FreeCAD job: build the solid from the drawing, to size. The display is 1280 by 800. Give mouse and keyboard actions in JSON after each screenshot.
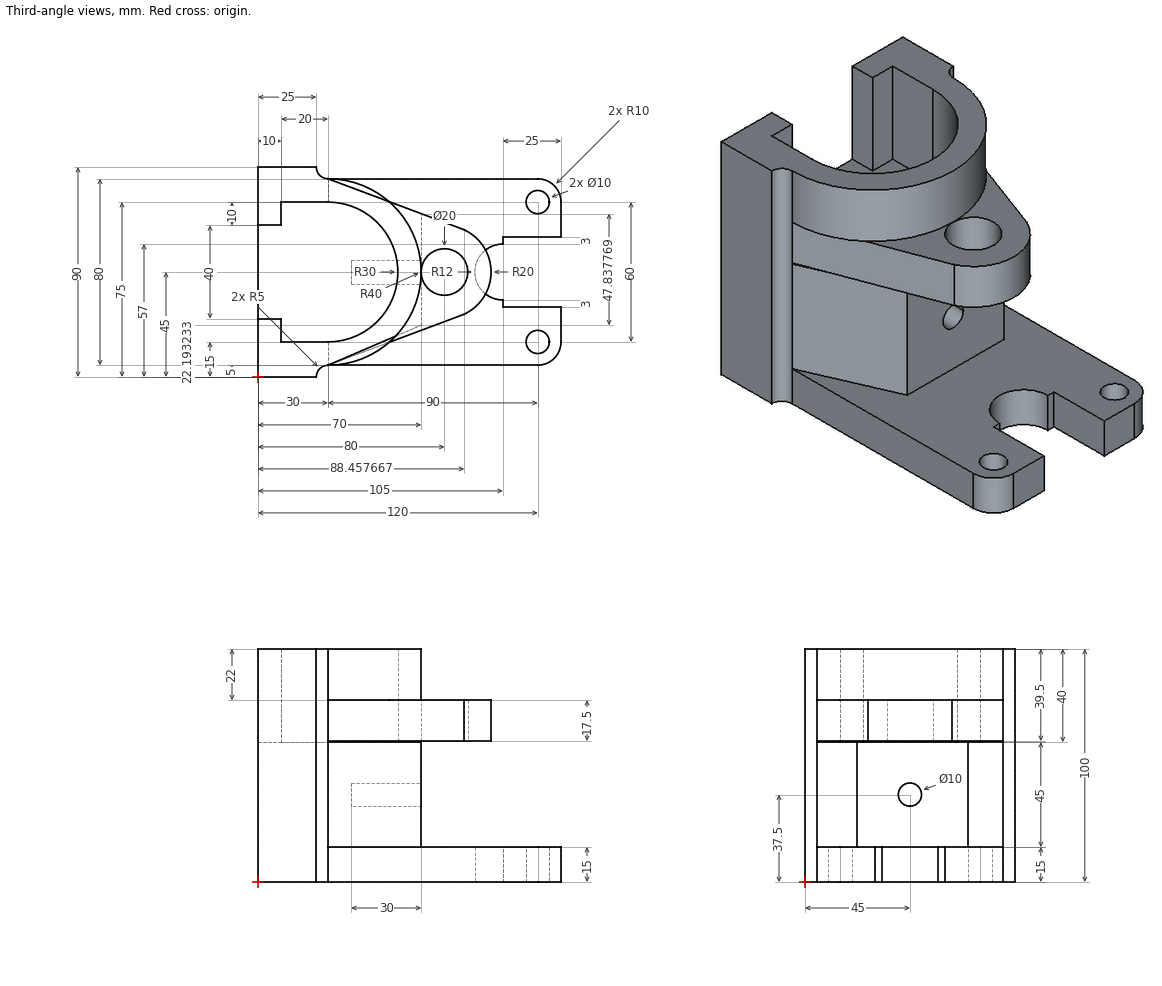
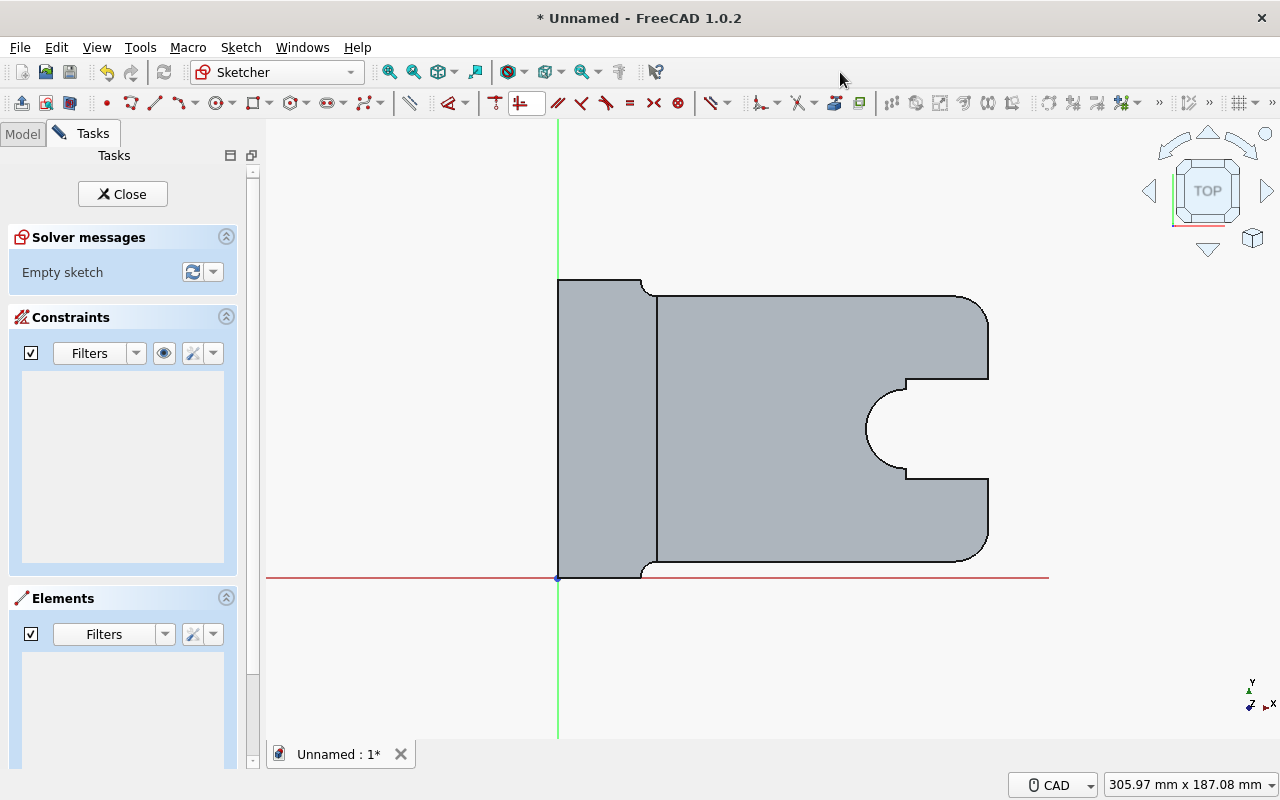
{"action": "scroll", "coordinate": [887, 479], "scroll_direction": "up", "scroll_amount": 2}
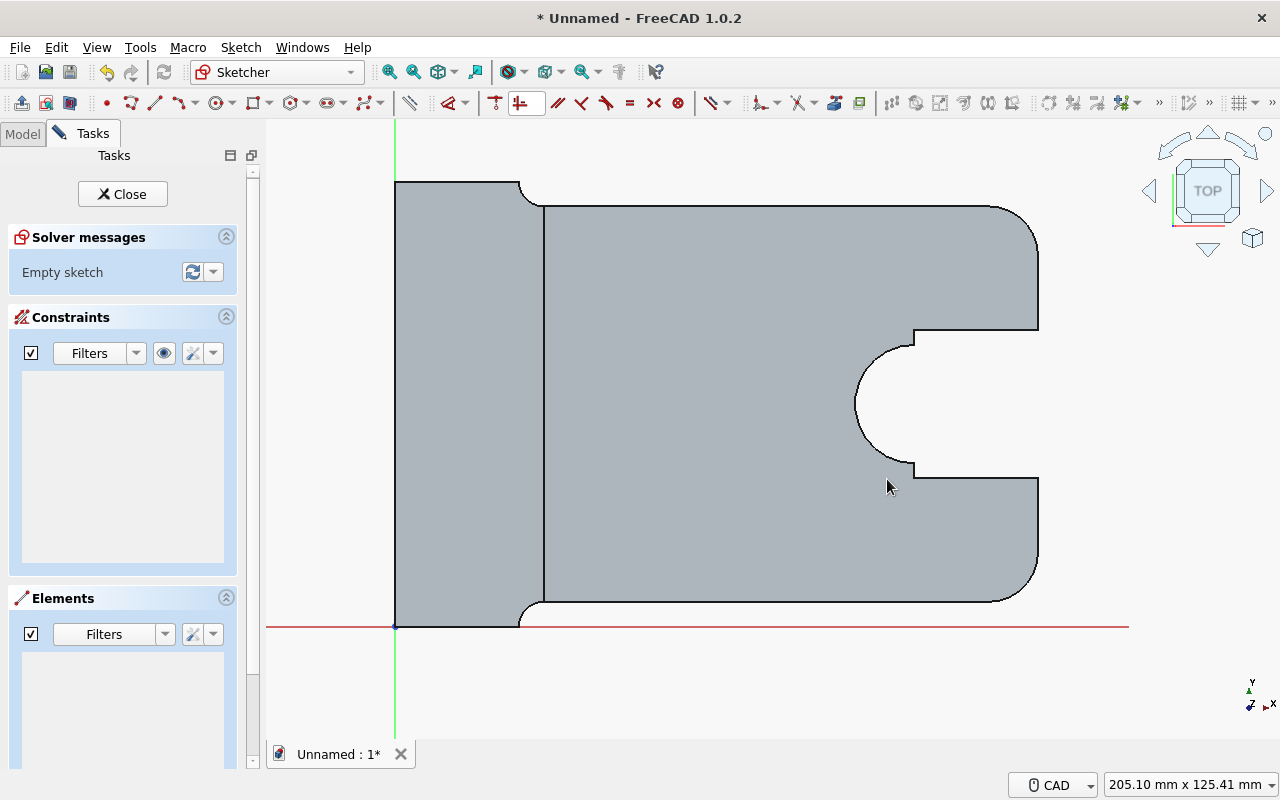
{"action": "left_click", "coordinate": [216, 104]}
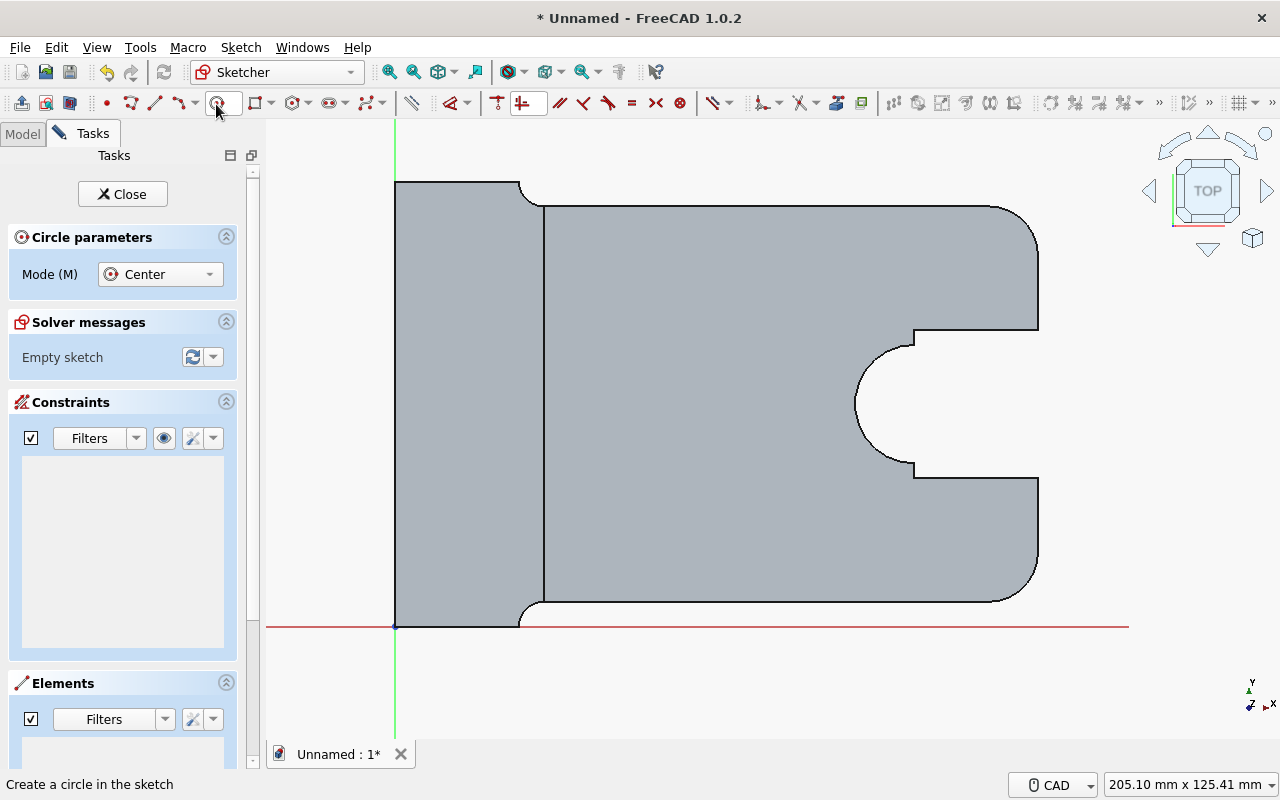
{"action": "left_click", "coordinate": [989, 256]}
{"action": "left_click", "coordinate": [1006, 238]}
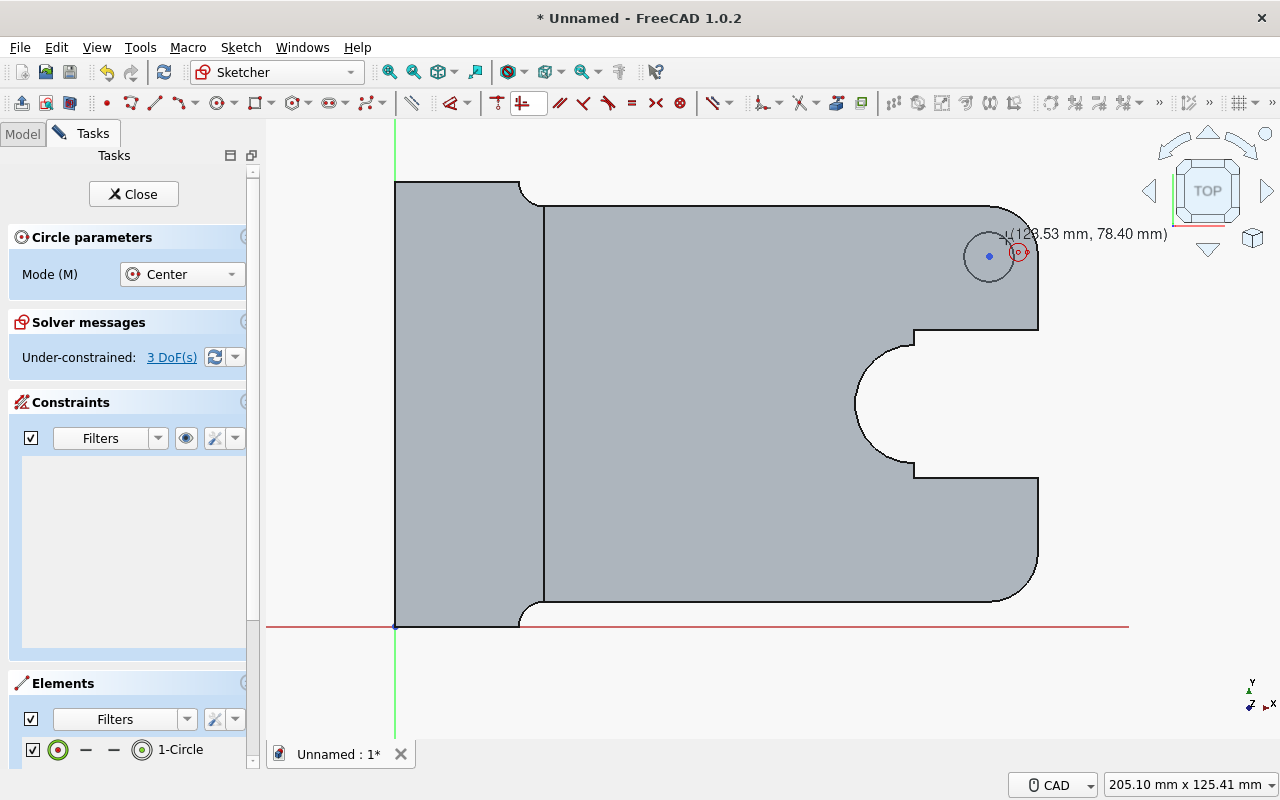
{"action": "left_click", "coordinate": [989, 552]}
{"action": "left_click", "coordinate": [1006, 535]}
{"action": "key", "text": "Escape"}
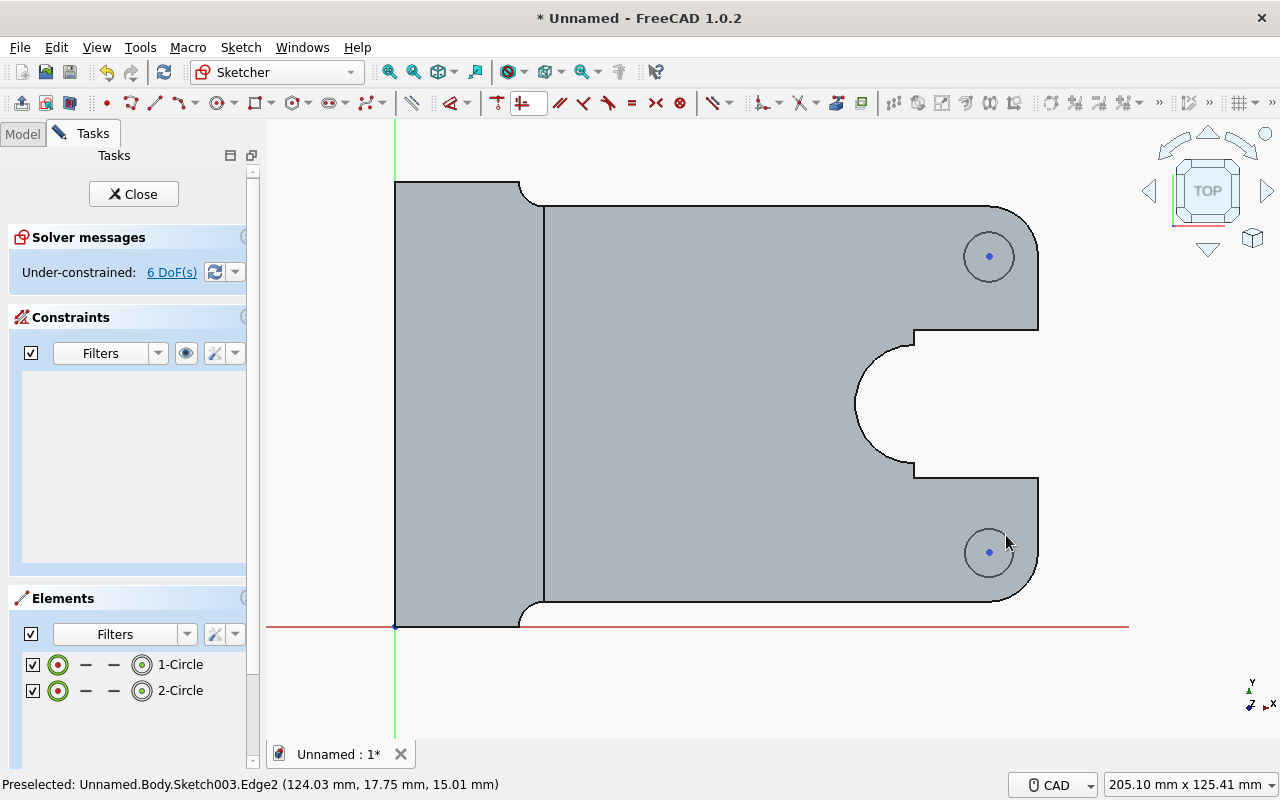
{"action": "left_click", "coordinate": [1006, 239]}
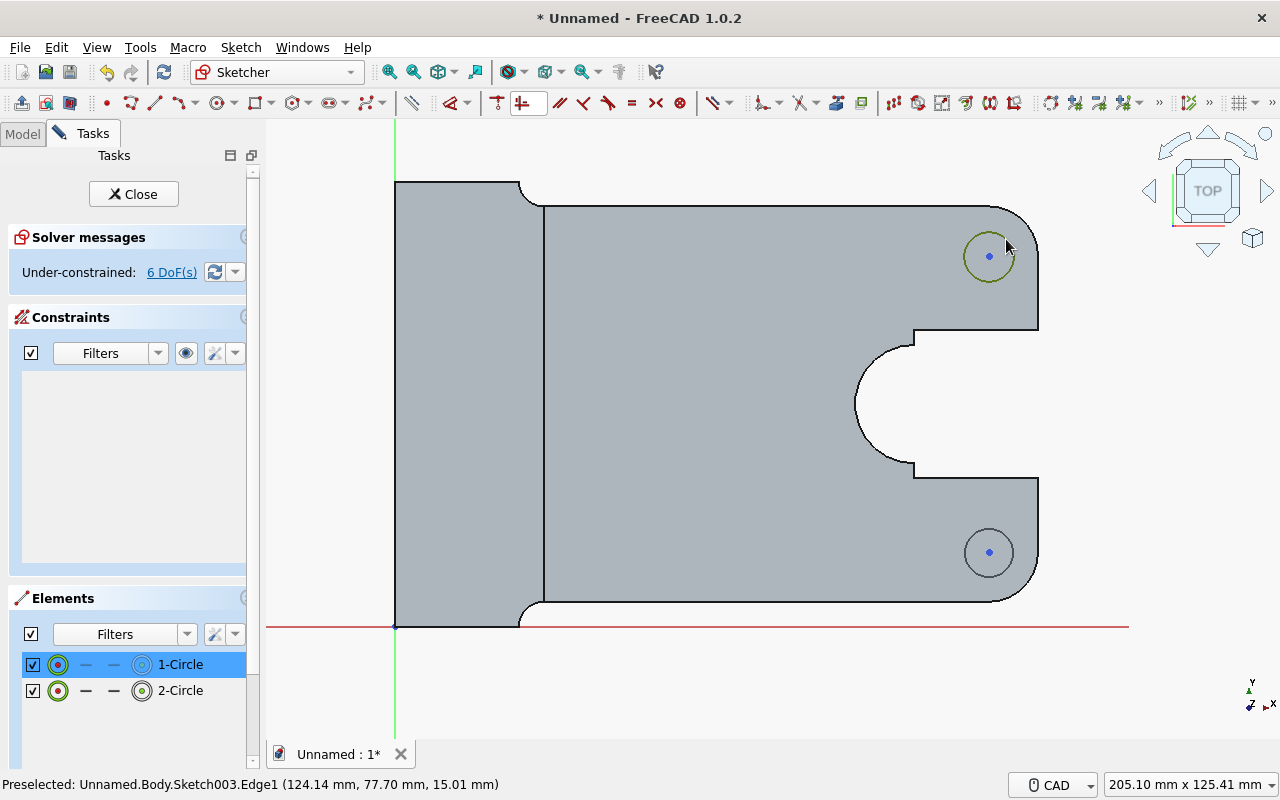
{"action": "left_click", "coordinate": [1006, 536]}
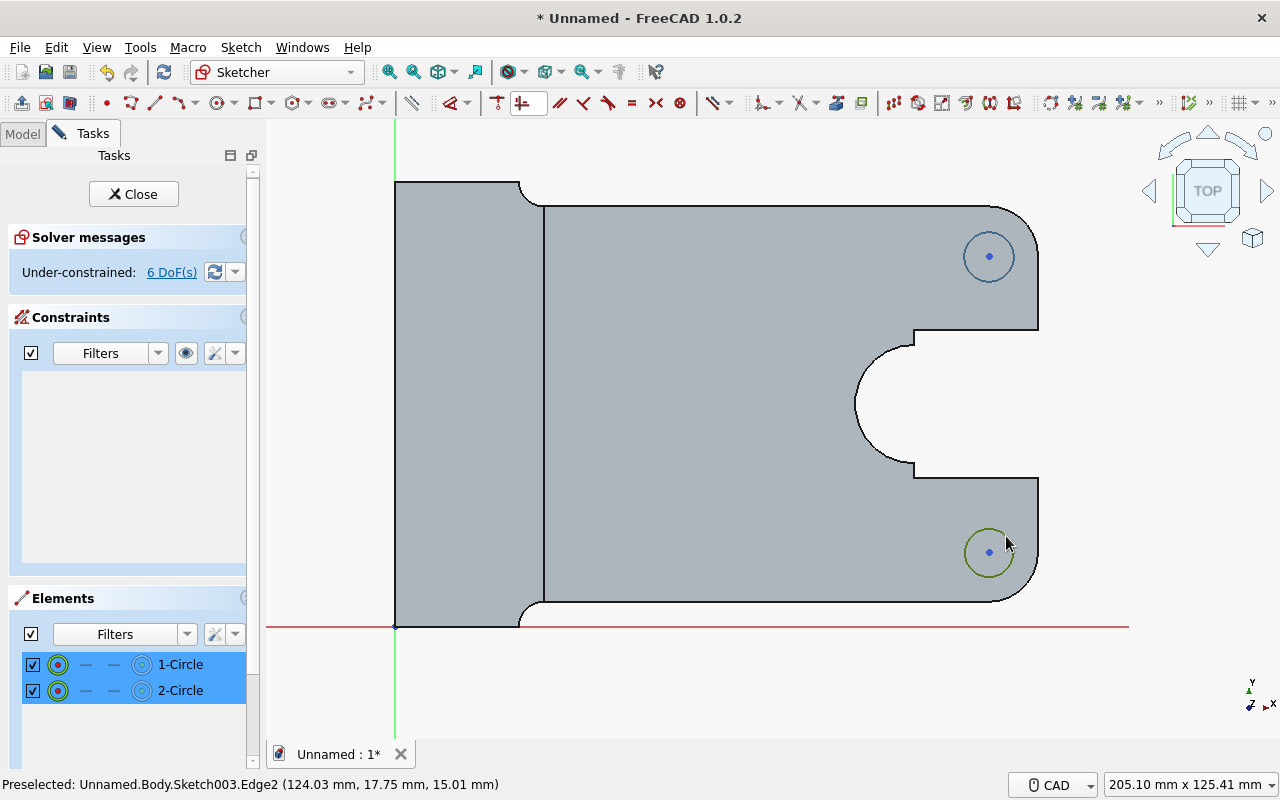
{"action": "left_click", "coordinate": [632, 104]}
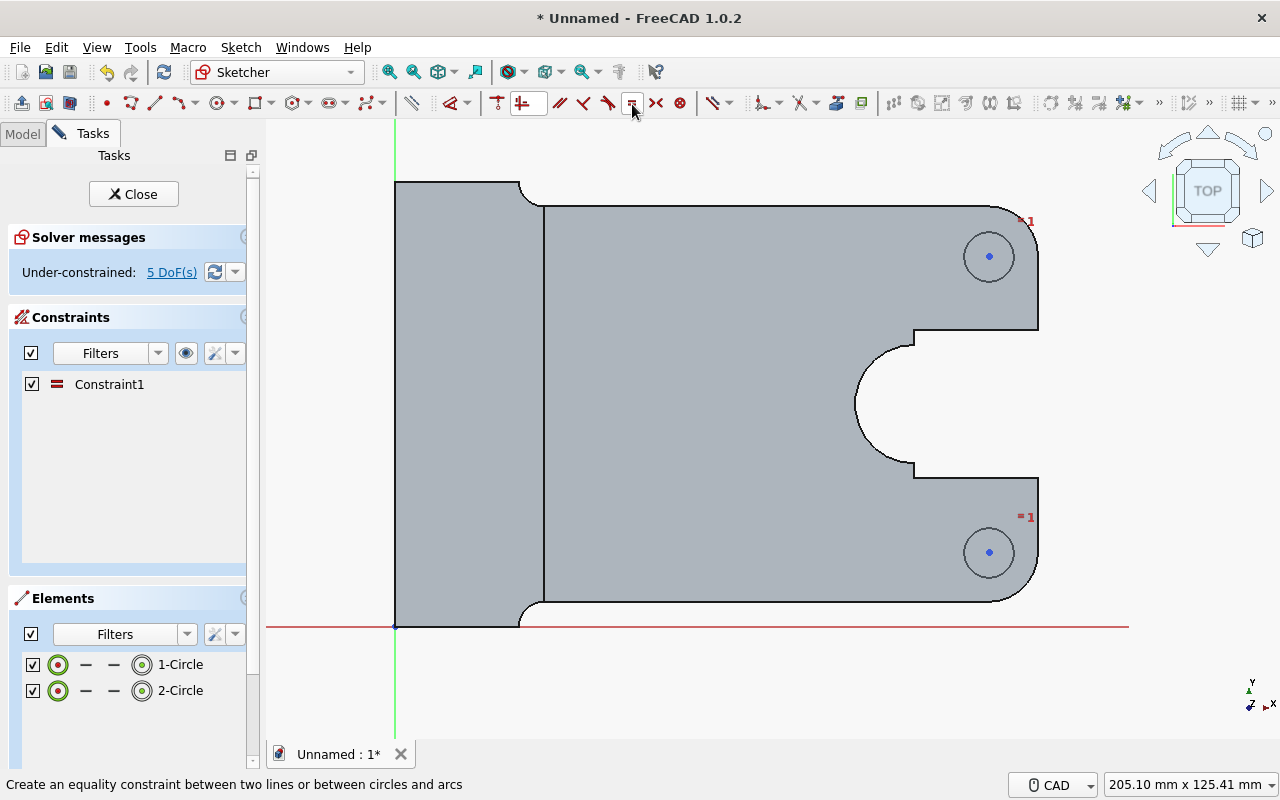
{"action": "left_click", "coordinate": [450, 104]}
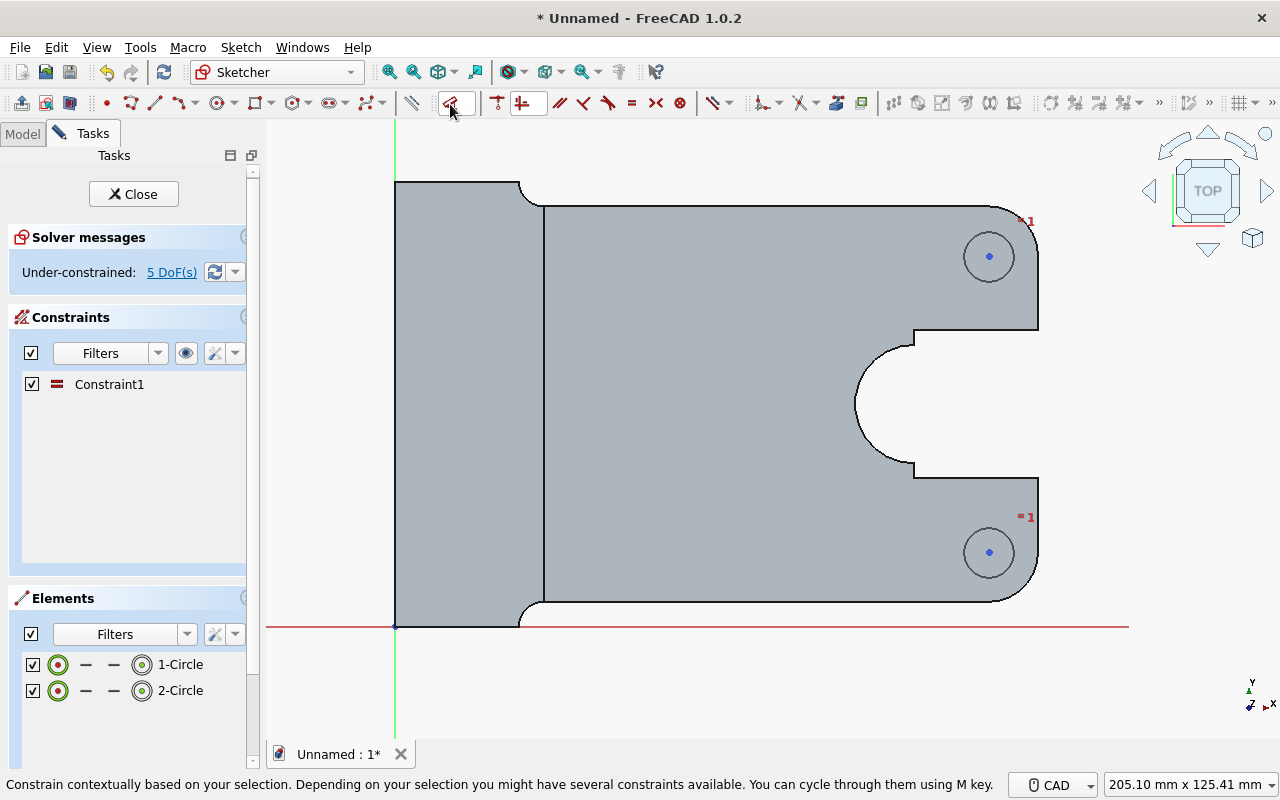
{"action": "left_click", "coordinate": [1006, 239]}
{"action": "left_click", "coordinate": [1028, 216]}